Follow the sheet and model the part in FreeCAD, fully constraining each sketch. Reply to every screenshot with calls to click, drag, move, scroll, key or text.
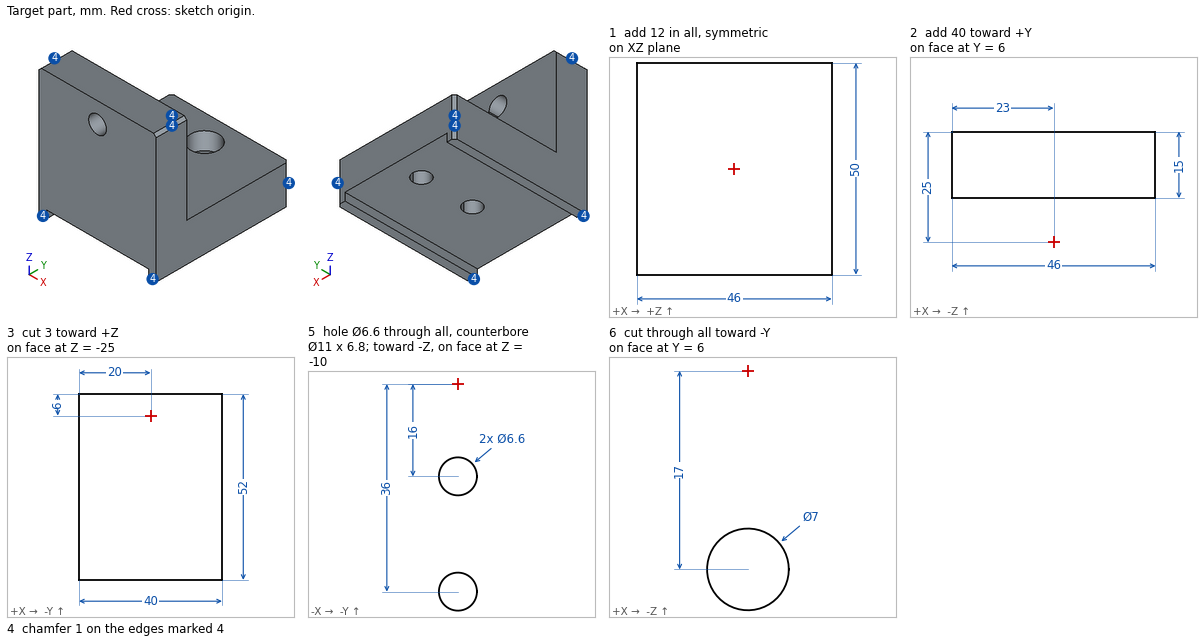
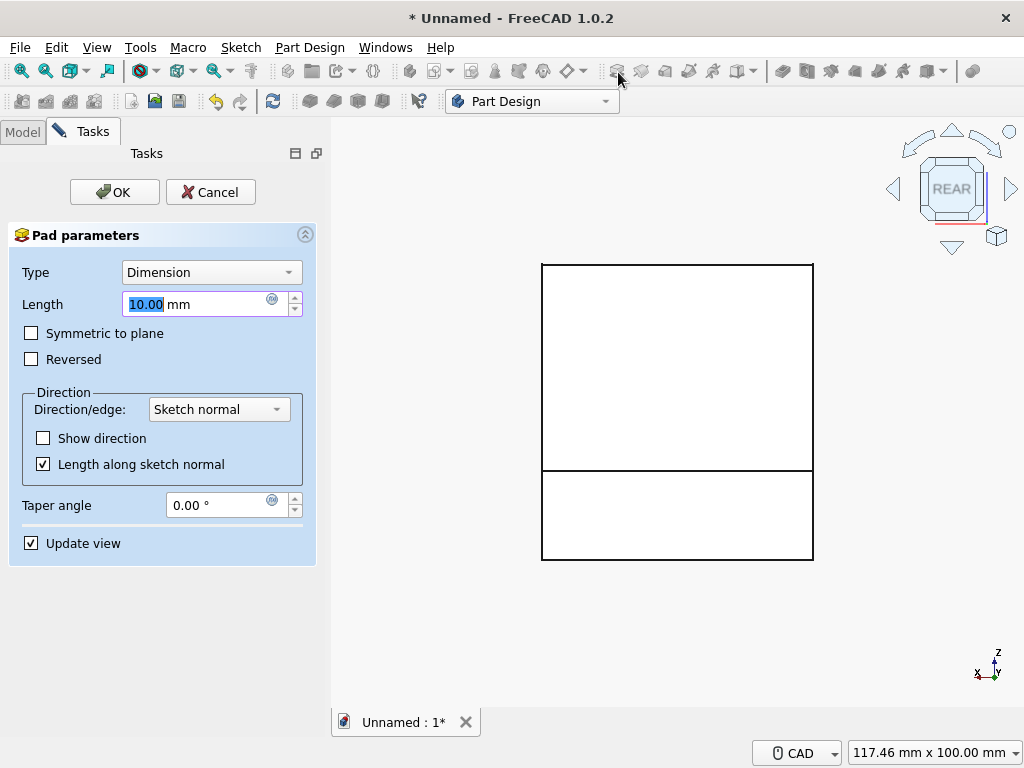
text(40)
key(Tab)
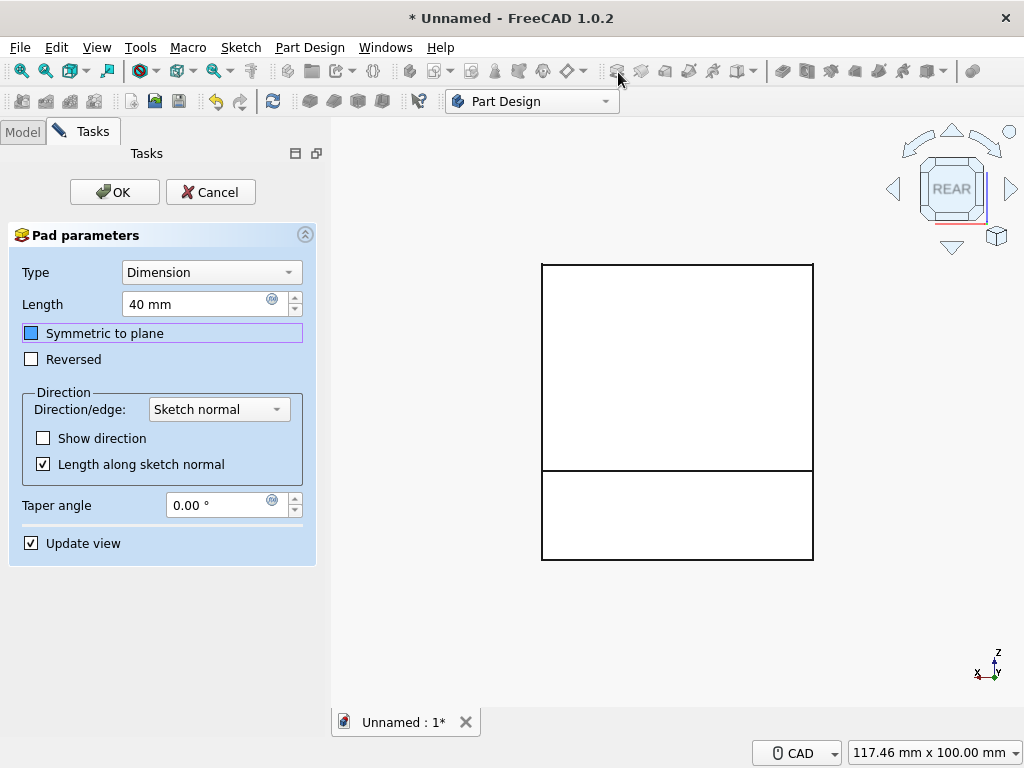
click(115, 192)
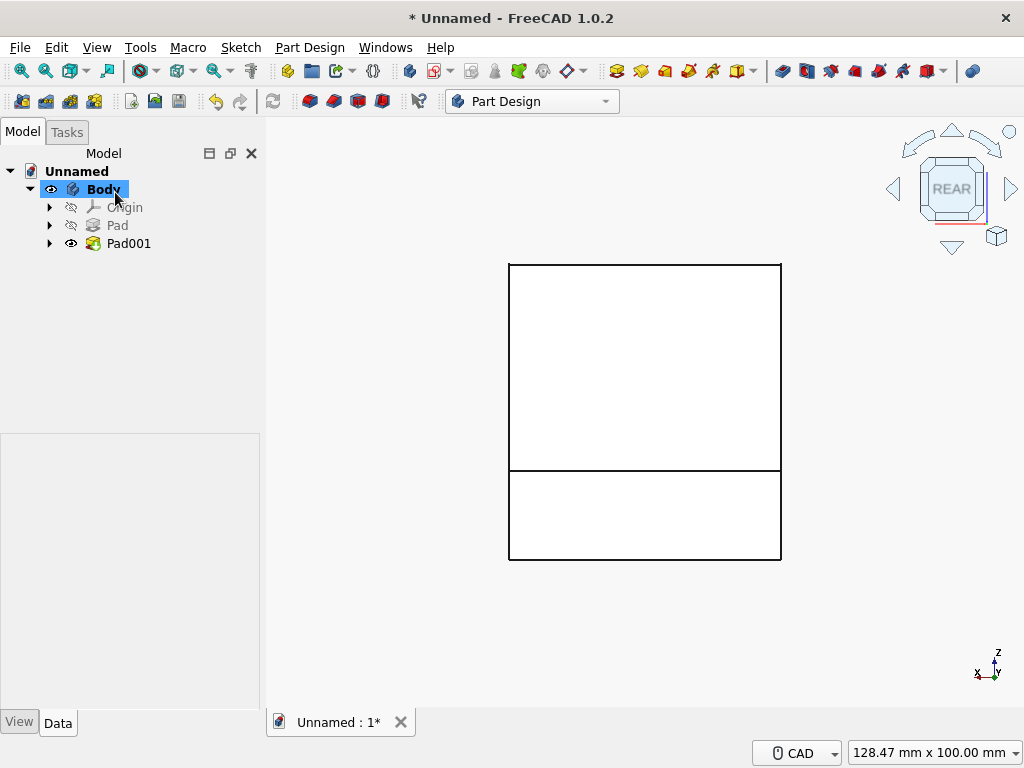
key(5)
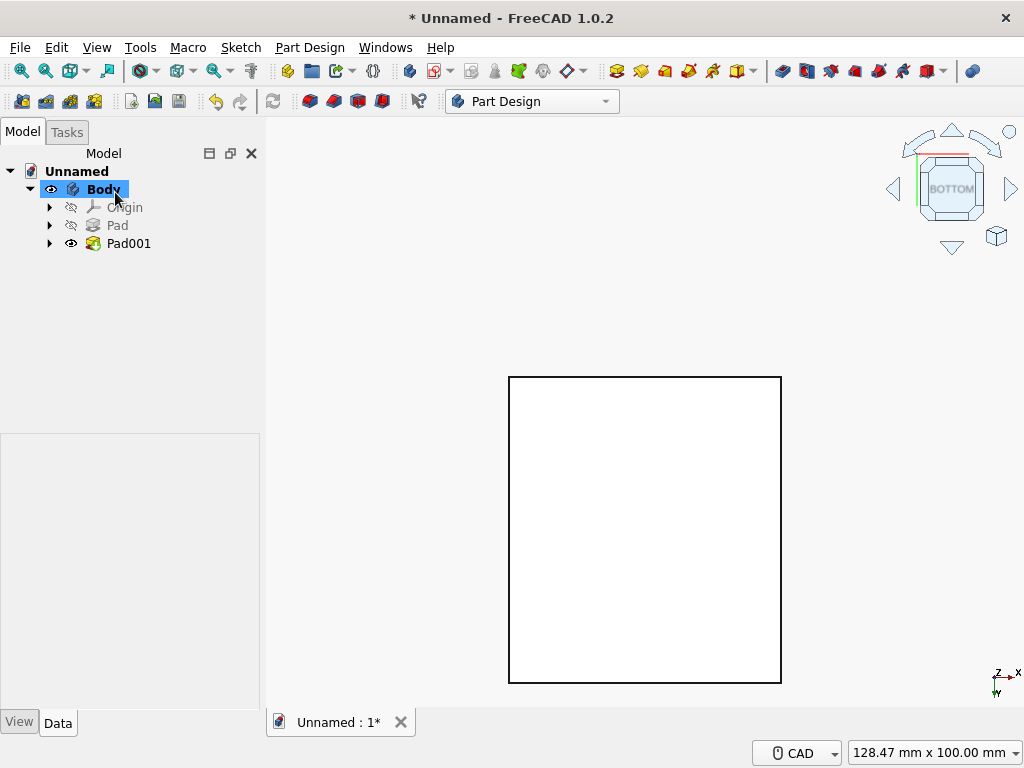
click(645, 529)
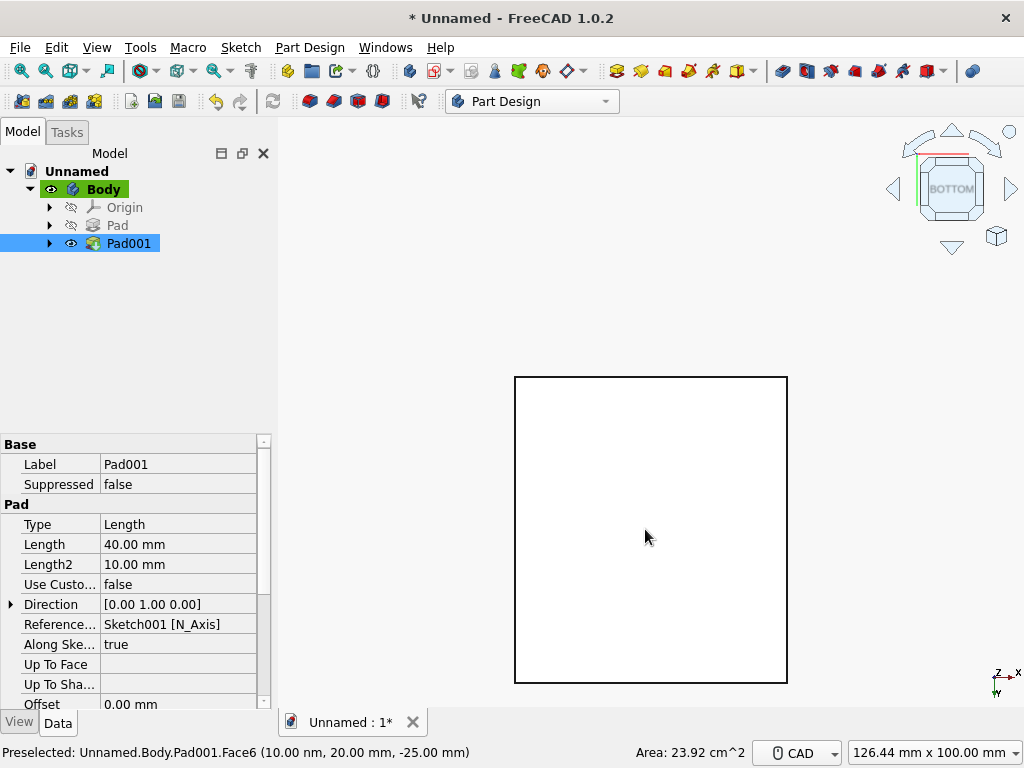
click(434, 72)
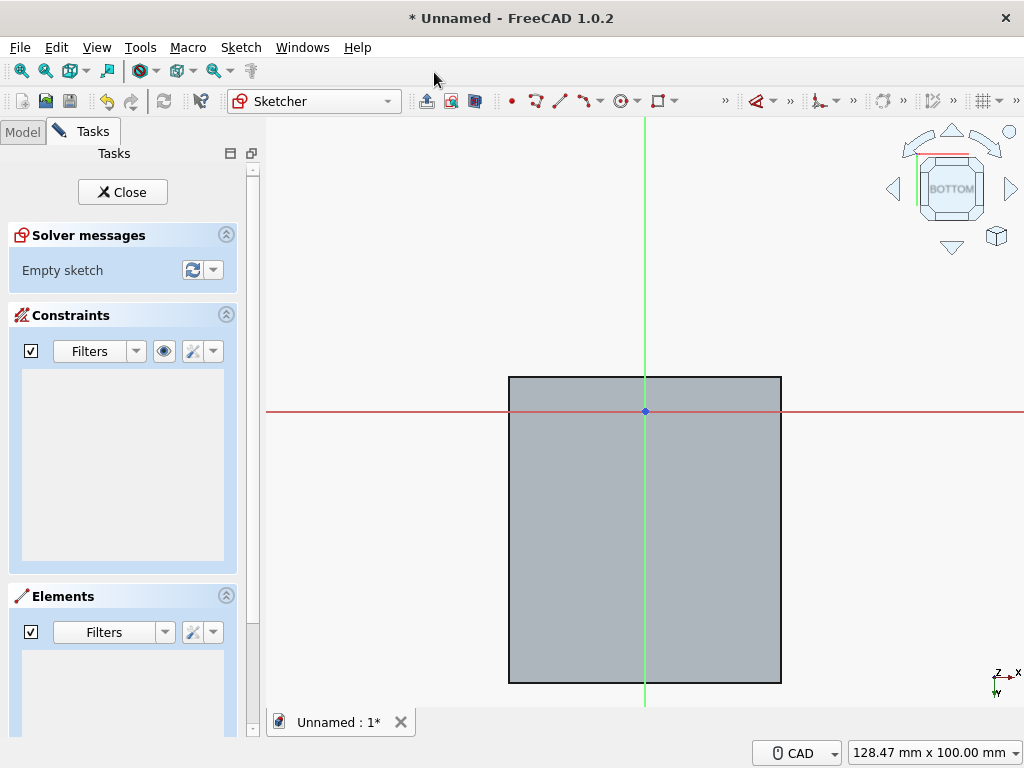
scroll(294, 145, down, 1)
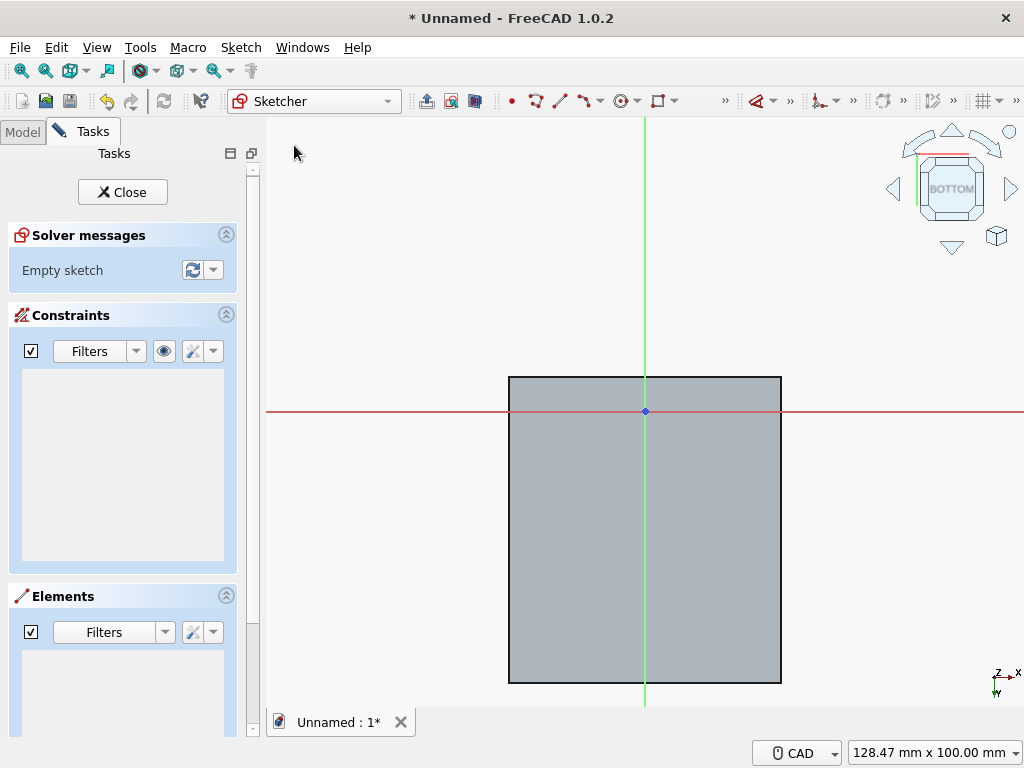
scroll(591, 558, up, 2)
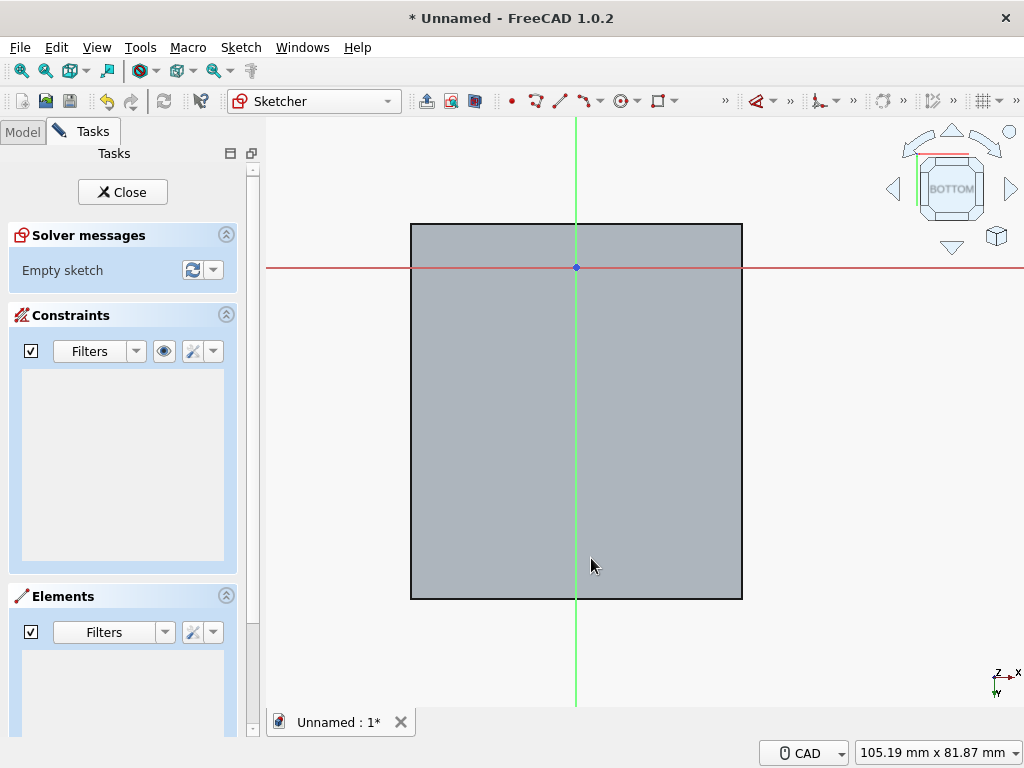
click(658, 102)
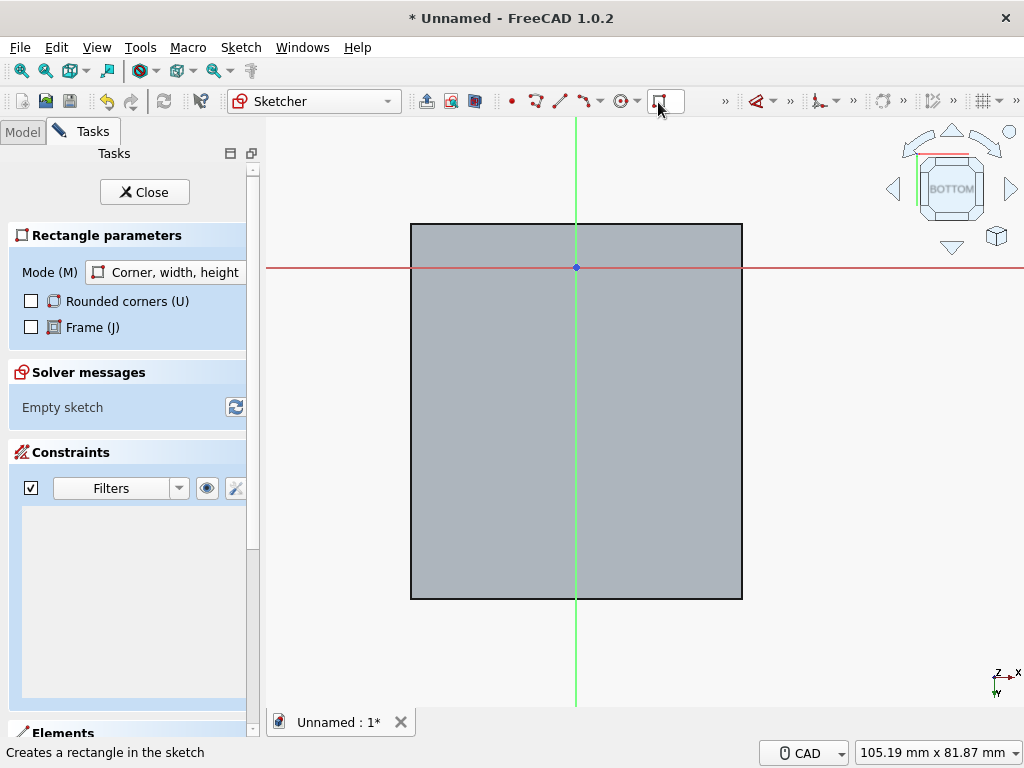
click(432, 224)
move(721, 599)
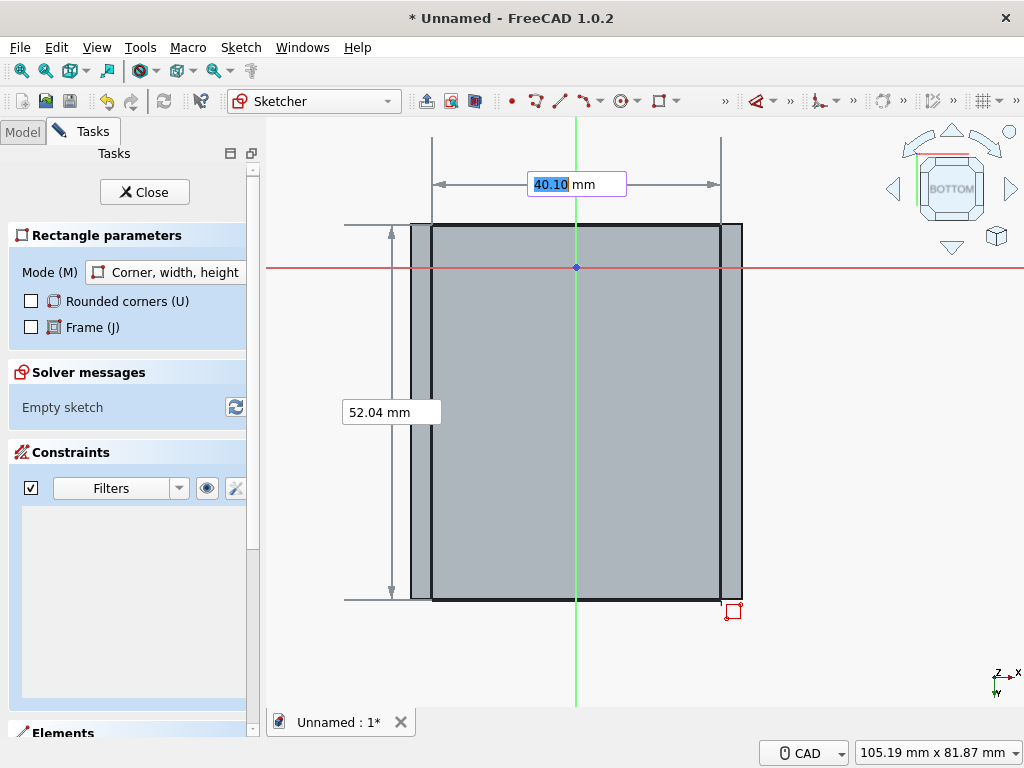
text(40)
key(Tab)
text(52)
key(Return)
key(Escape)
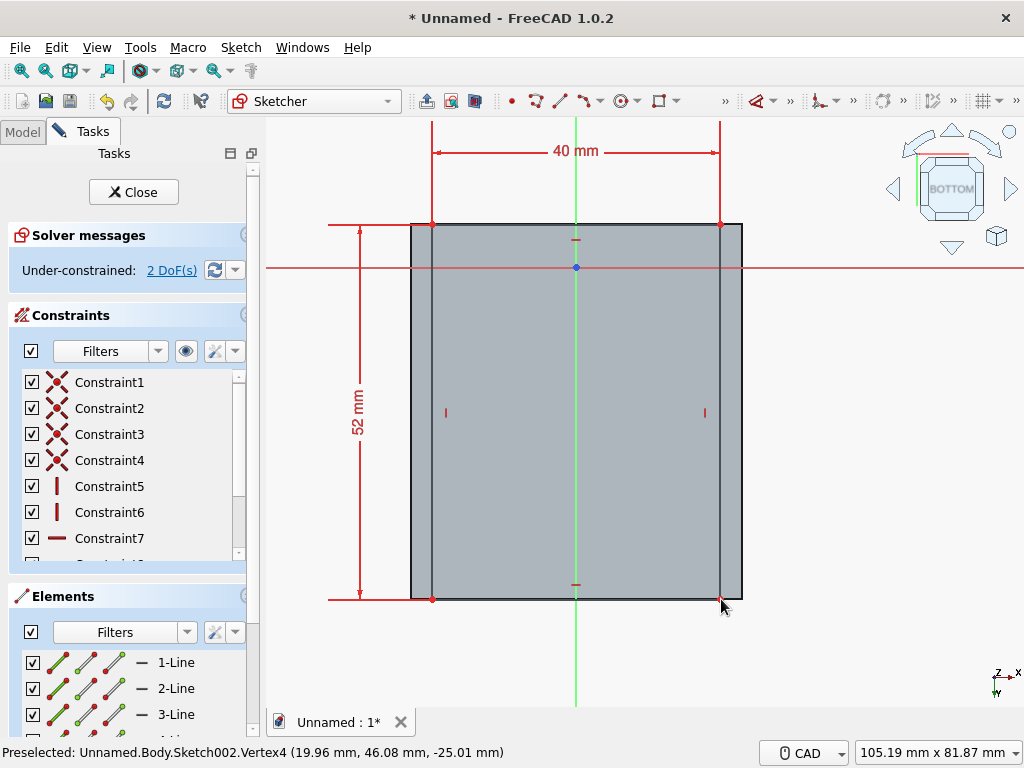
click(756, 102)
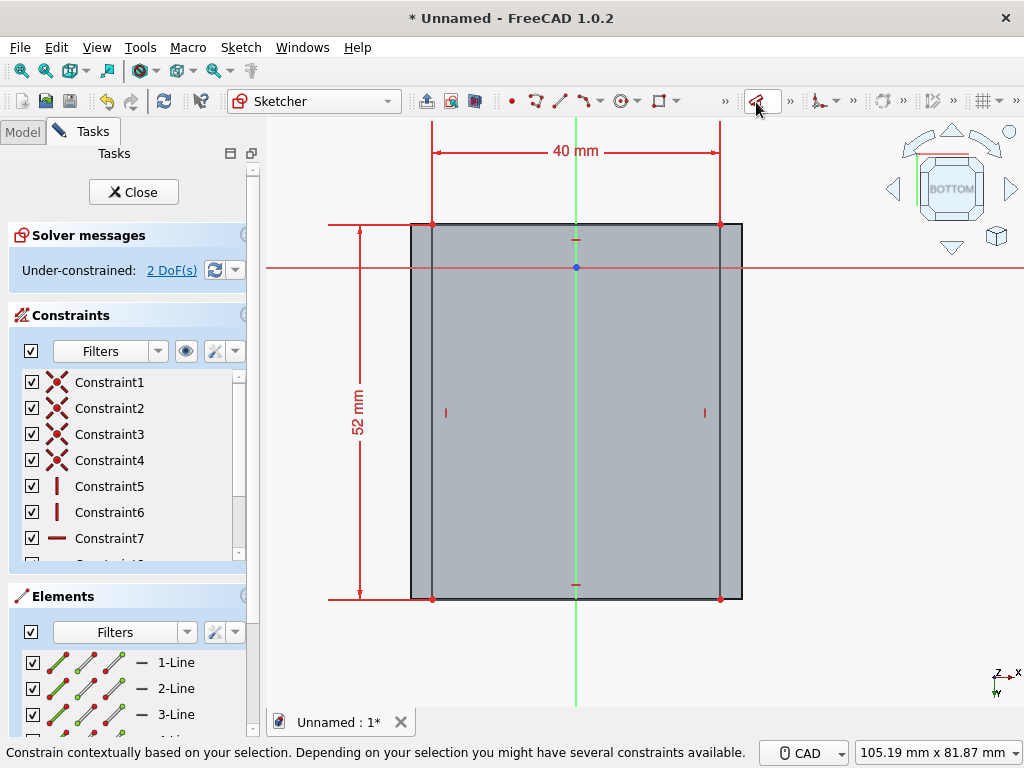
click(432, 225)
click(398, 246)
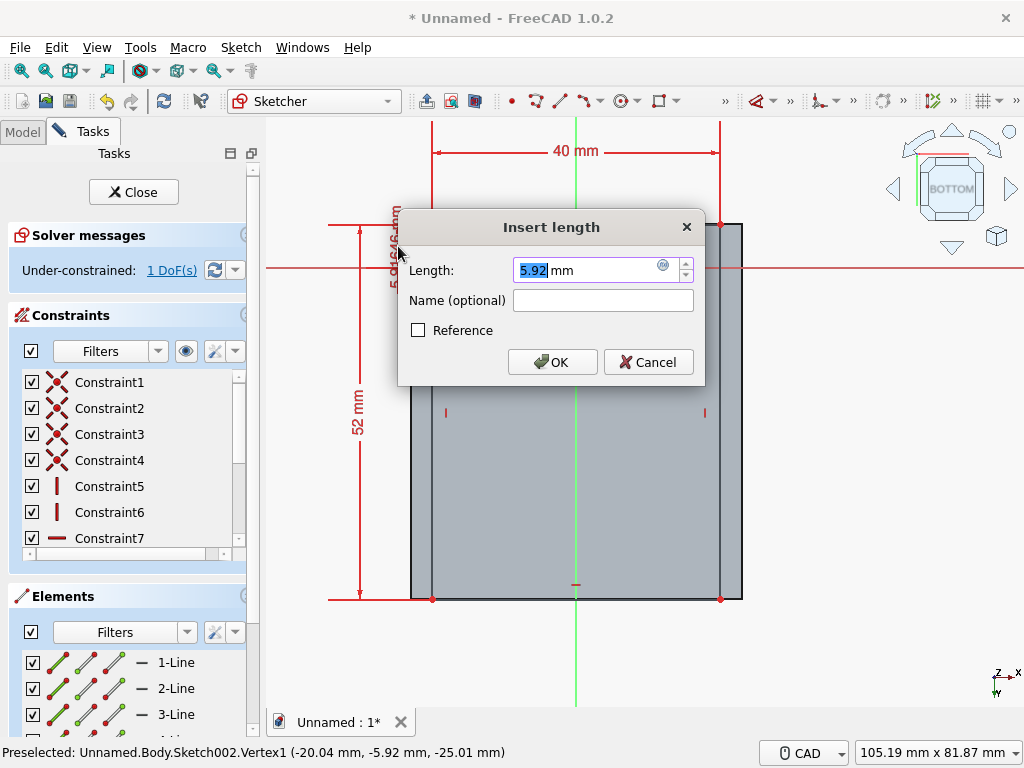
text(6)
key(Return)